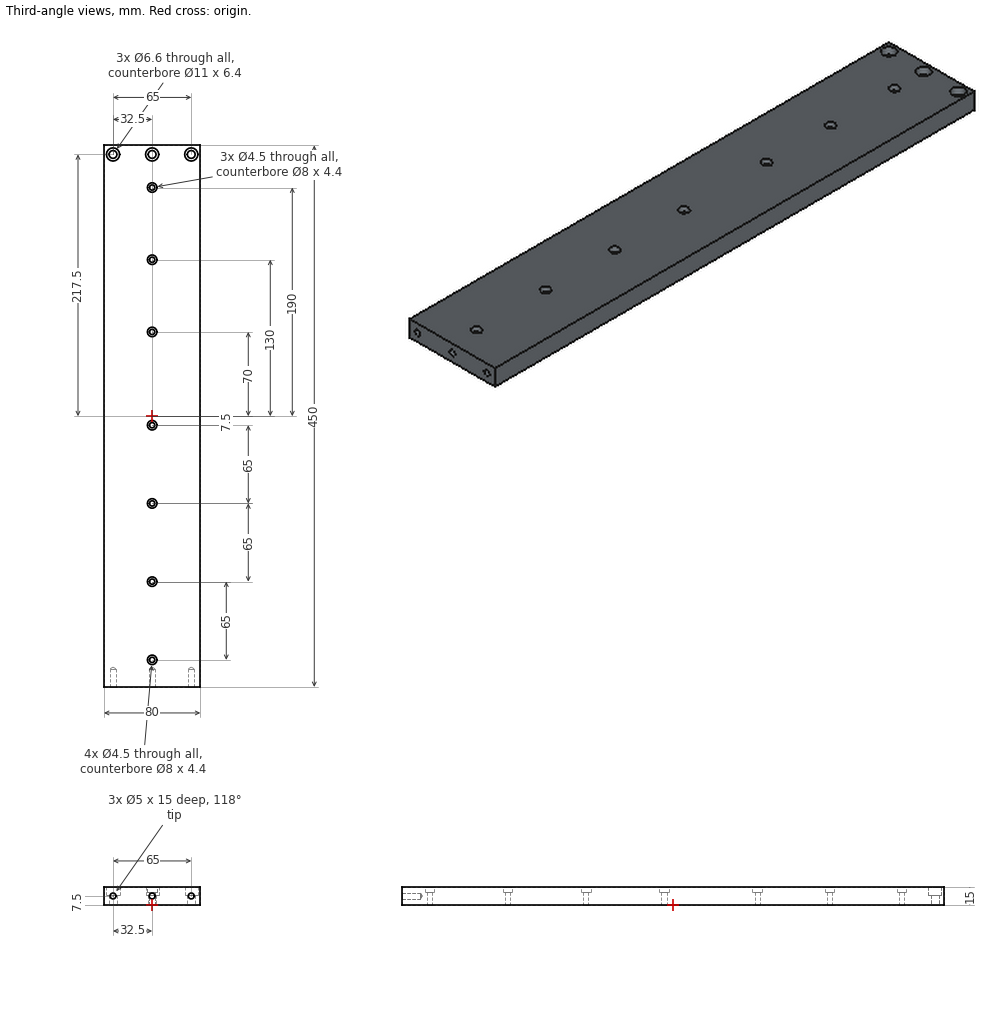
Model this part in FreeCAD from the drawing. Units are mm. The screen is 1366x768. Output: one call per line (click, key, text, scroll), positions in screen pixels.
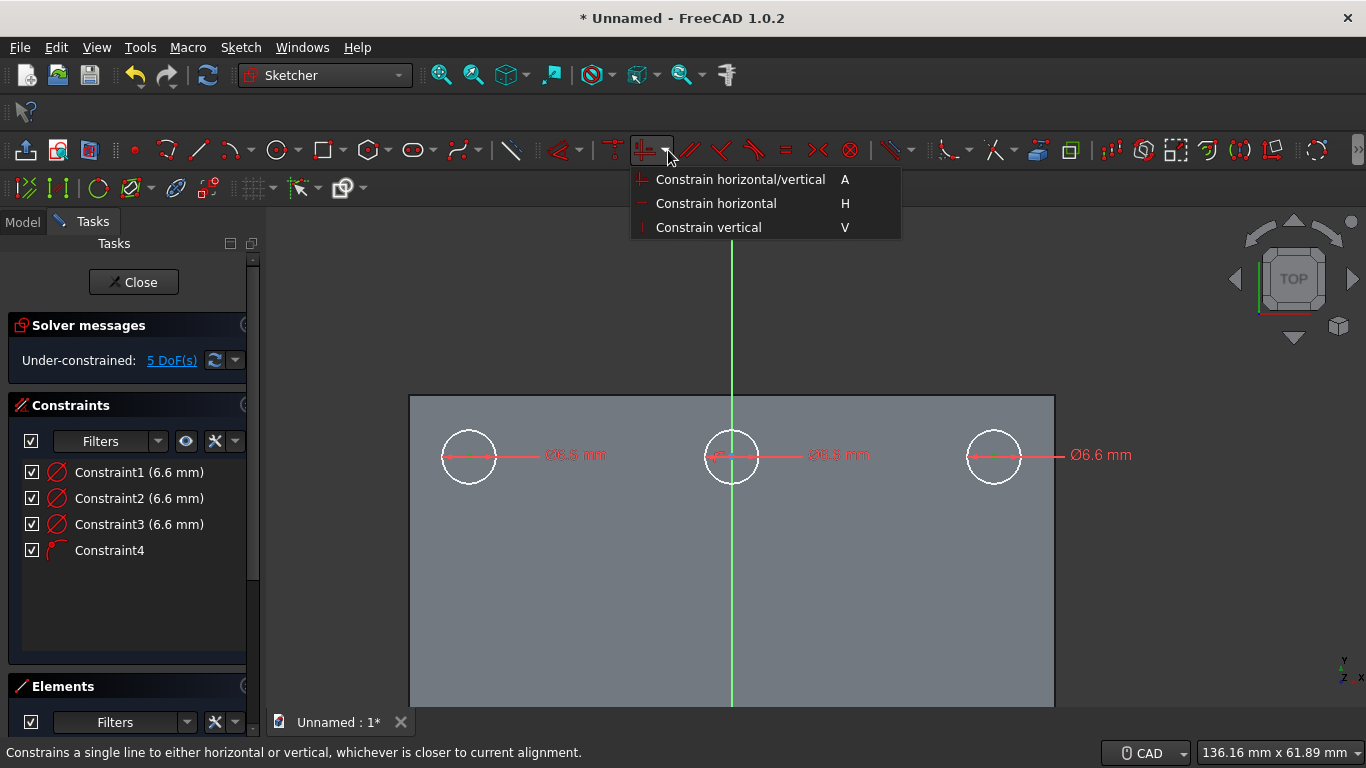
click(766, 203)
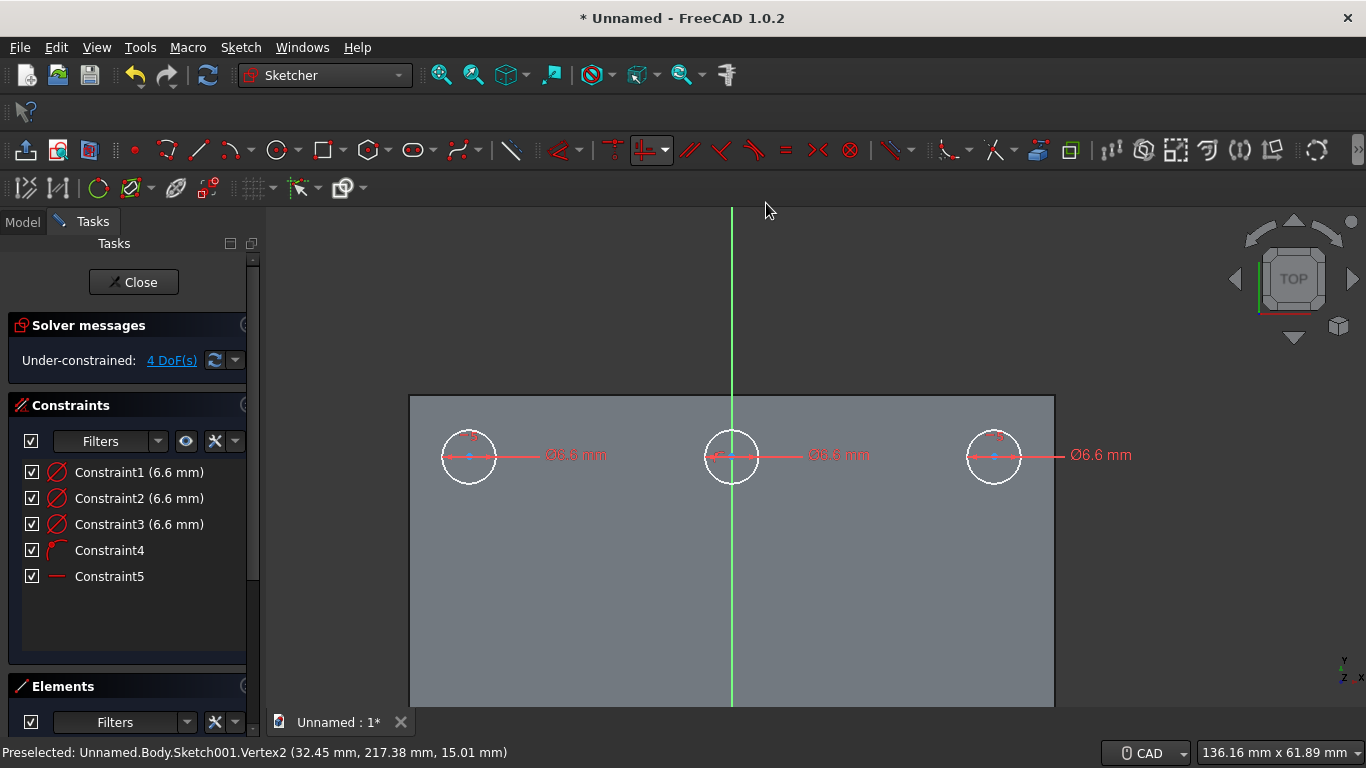
click(469, 457)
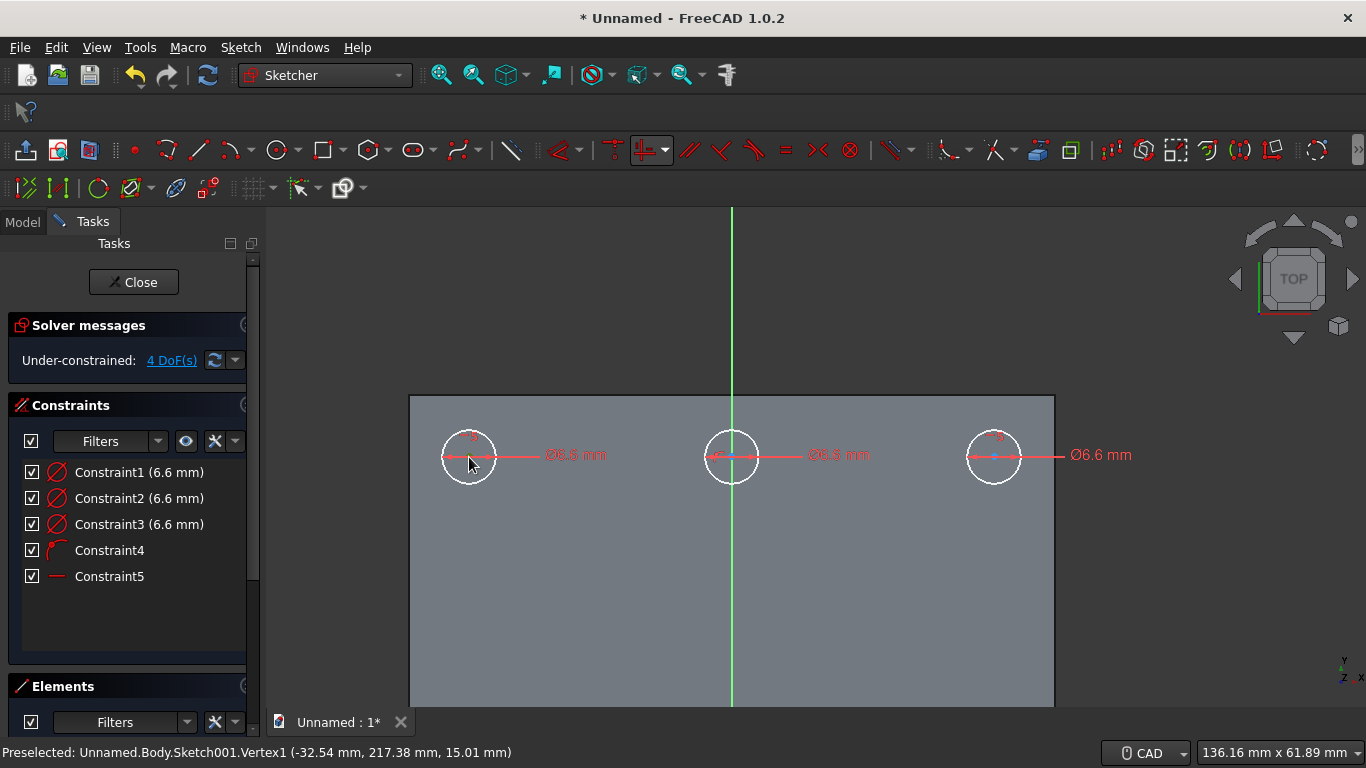
click(732, 457)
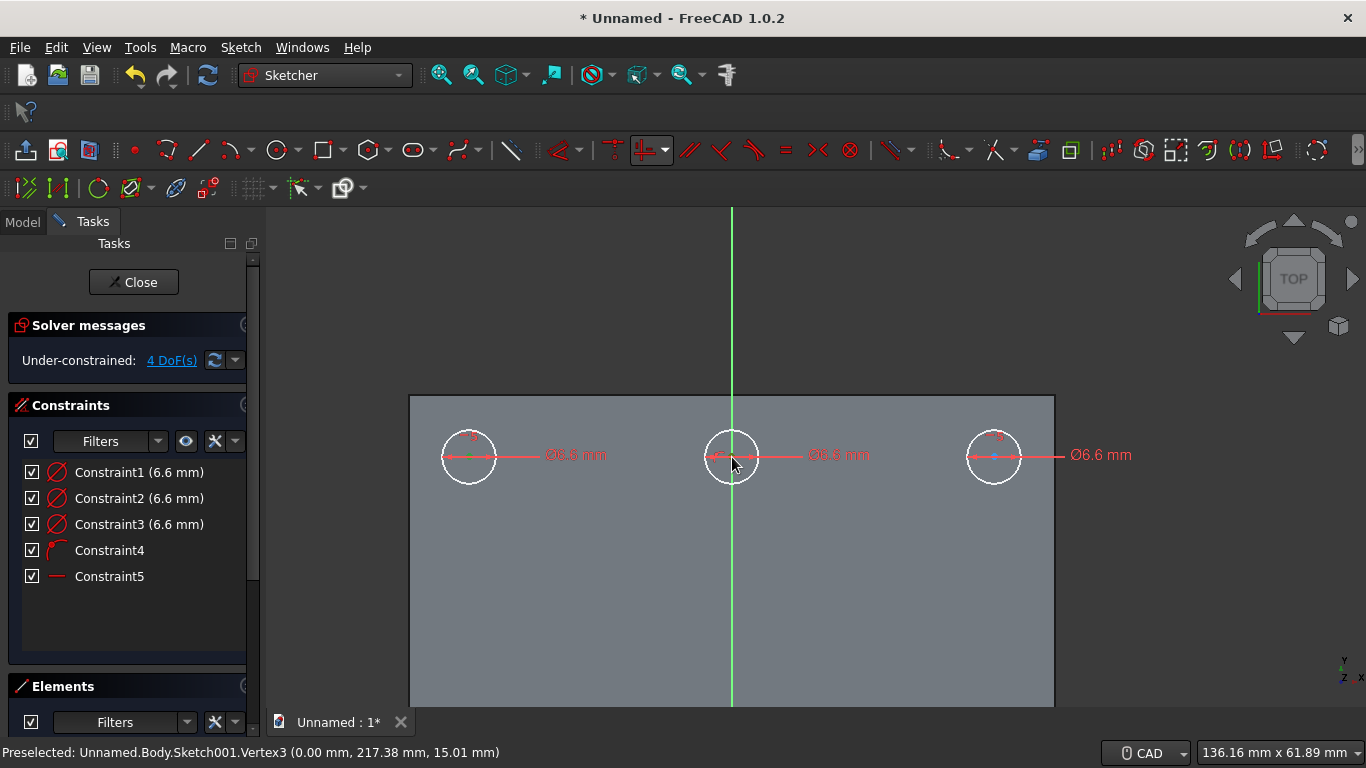
click(668, 150)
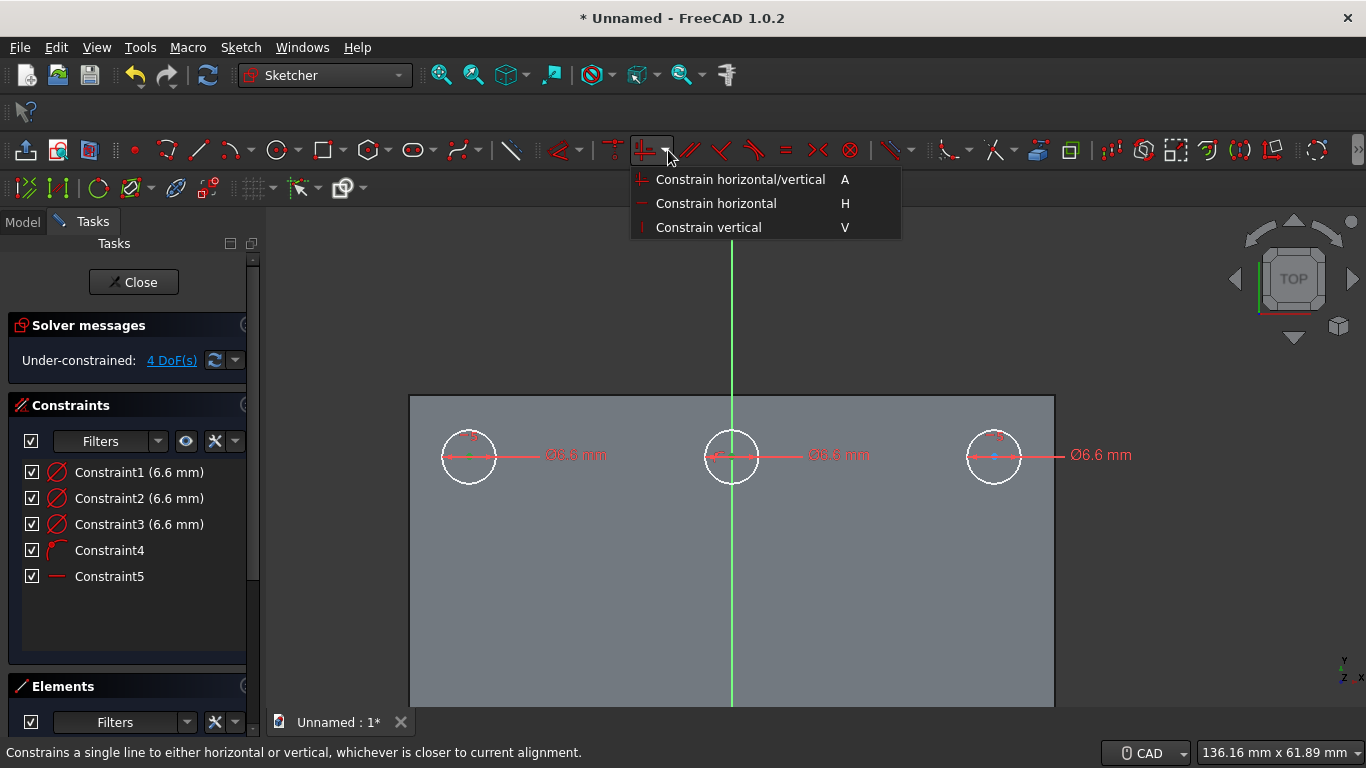
click(766, 203)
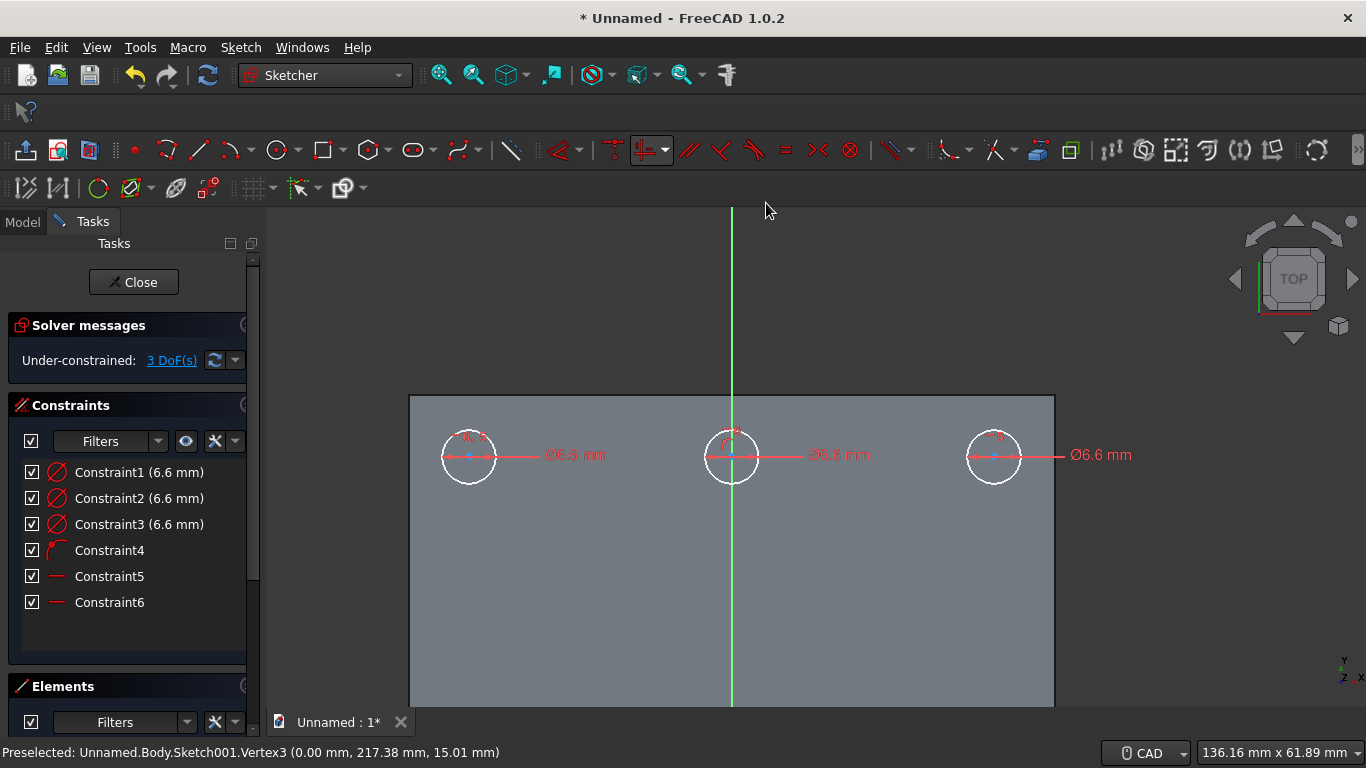
click(558, 150)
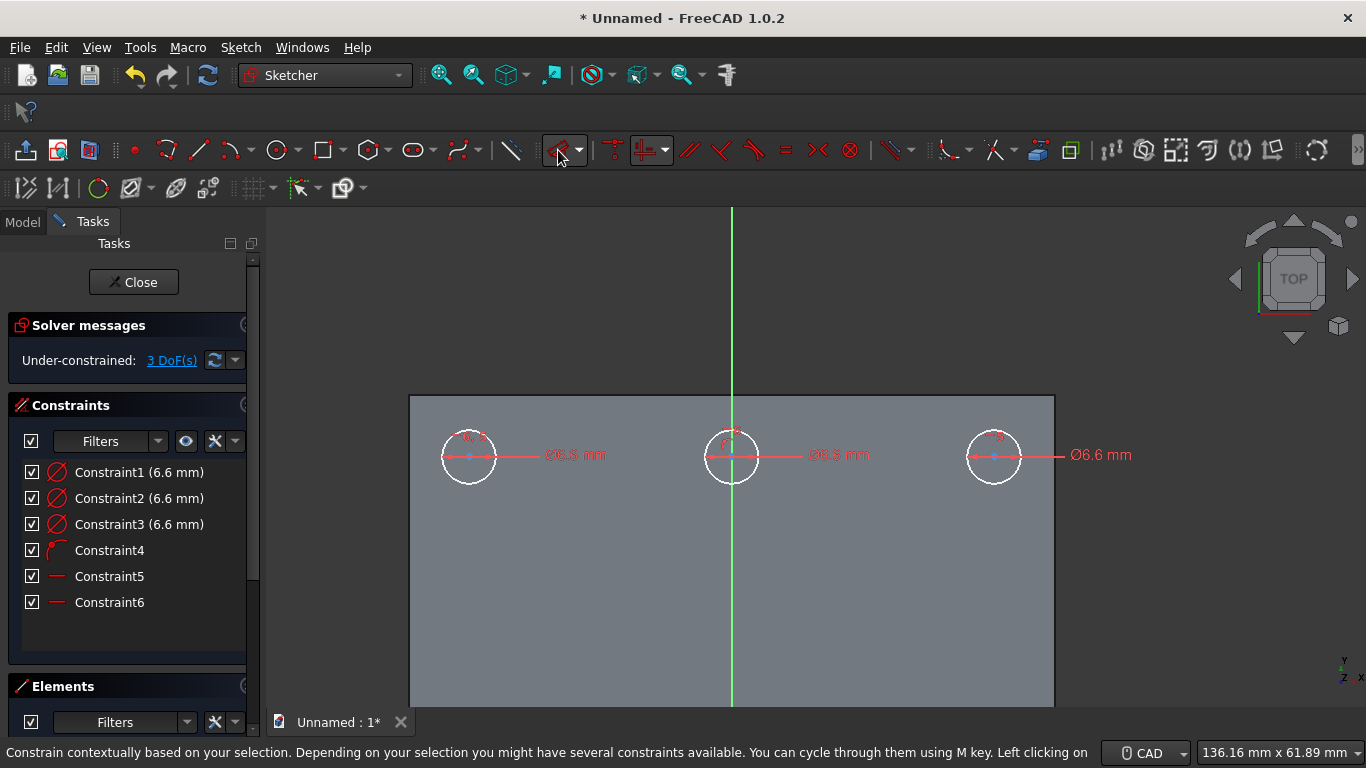
click(469, 457)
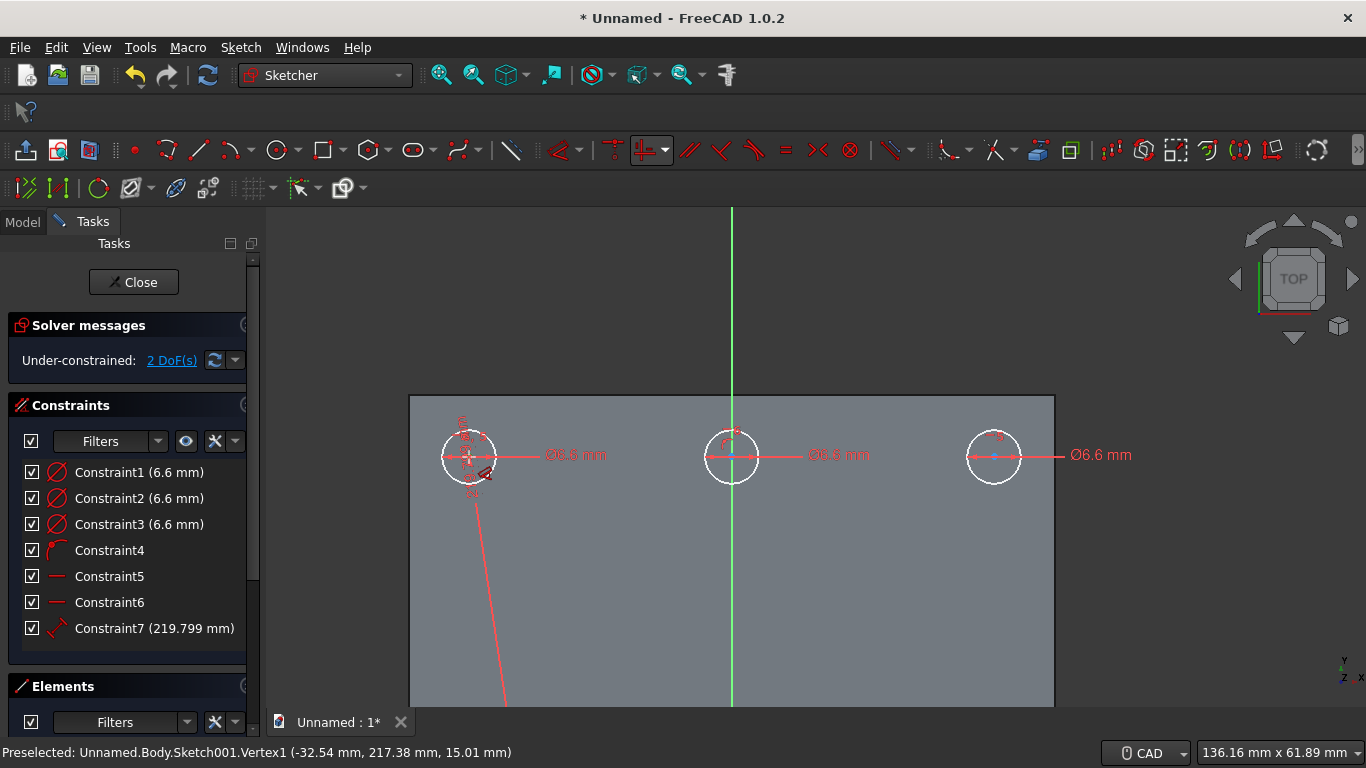
click(994, 457)
click(611, 491)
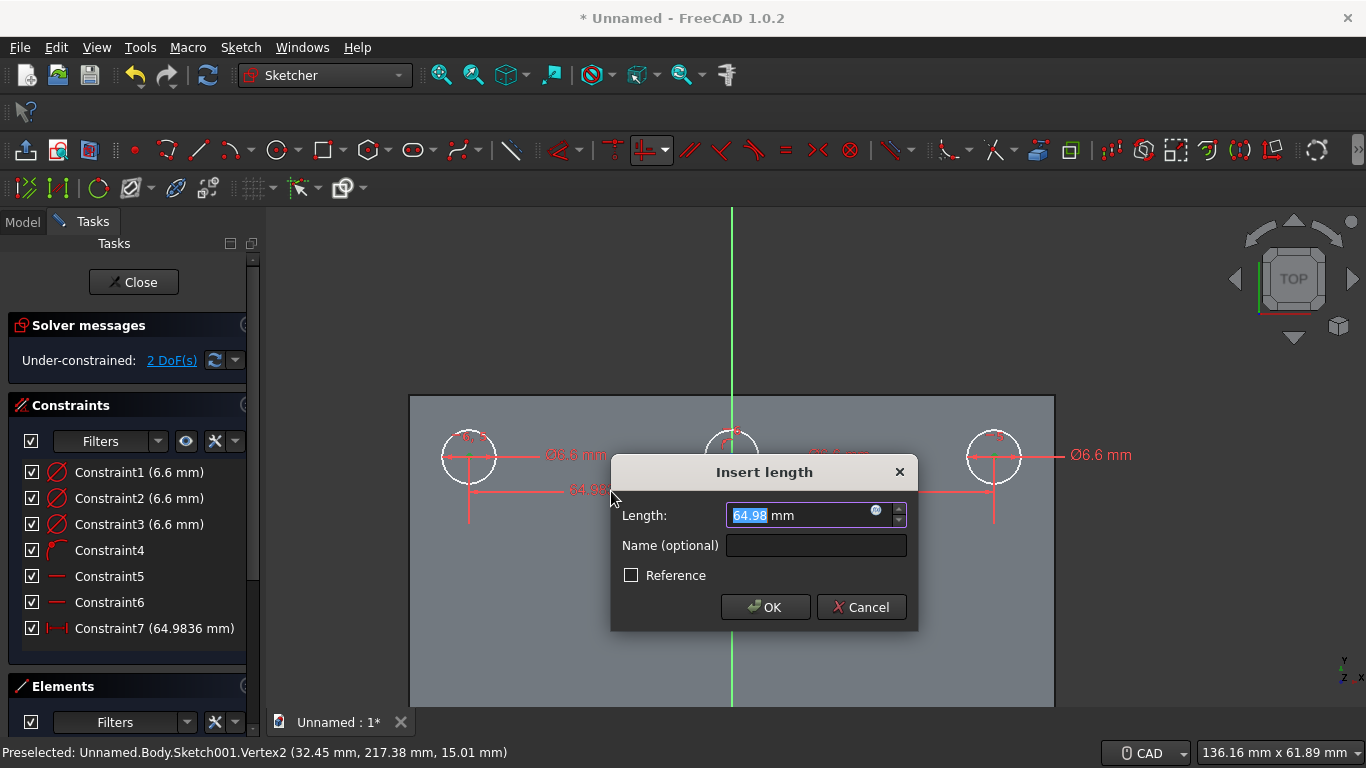
text(65)
key(Return)